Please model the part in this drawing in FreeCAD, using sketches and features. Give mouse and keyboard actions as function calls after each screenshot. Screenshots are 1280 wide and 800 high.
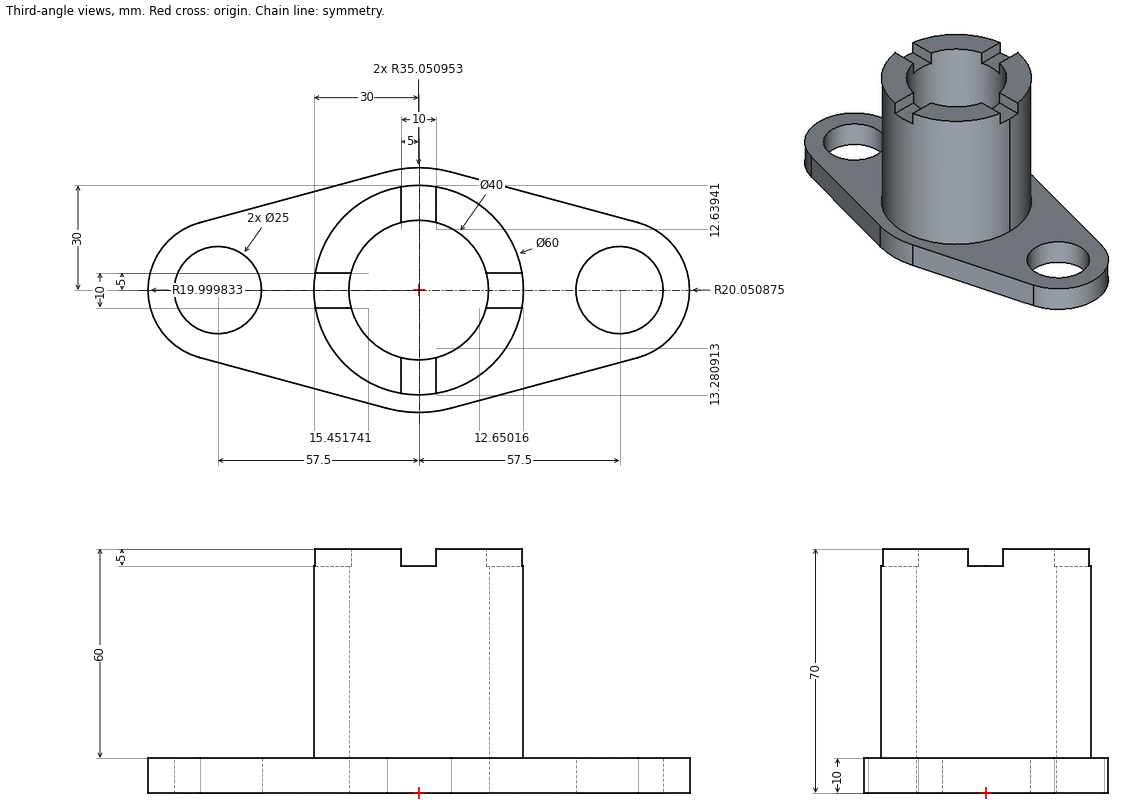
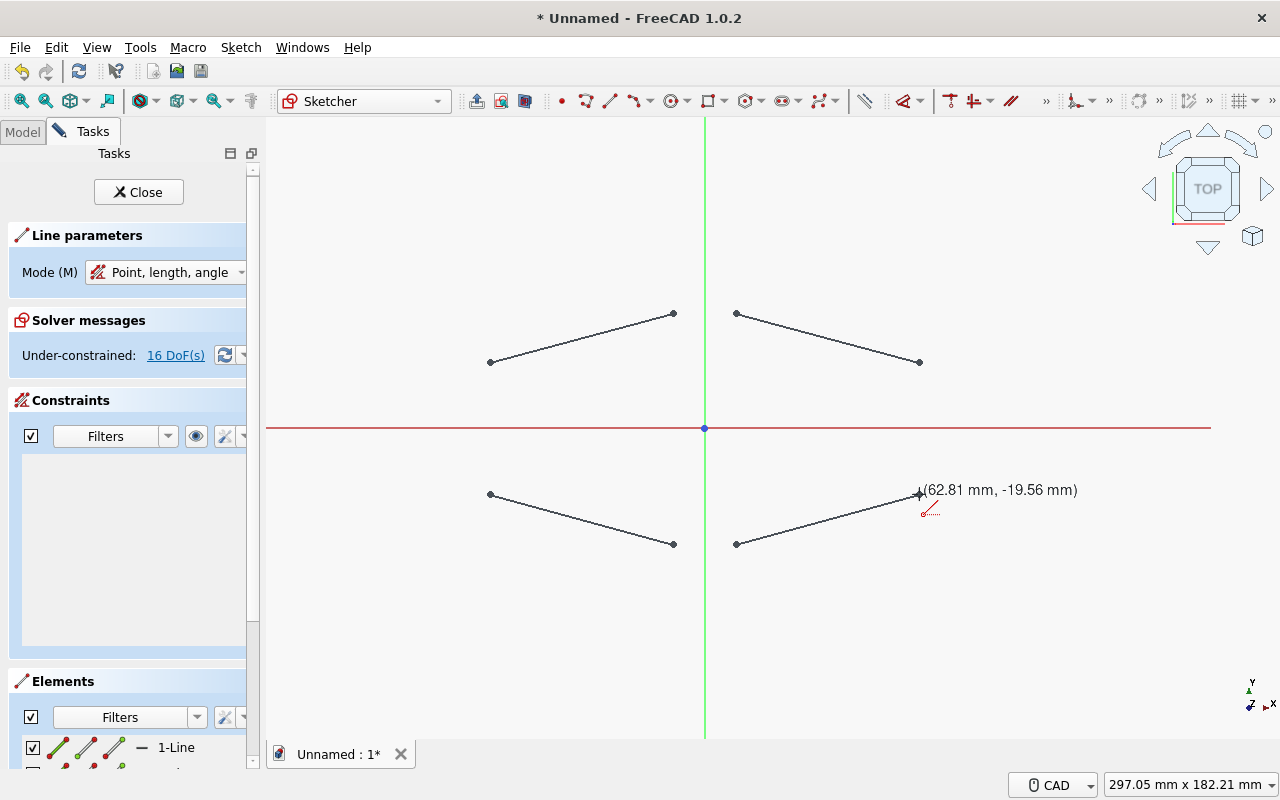
key(g)
key(3)
key(a)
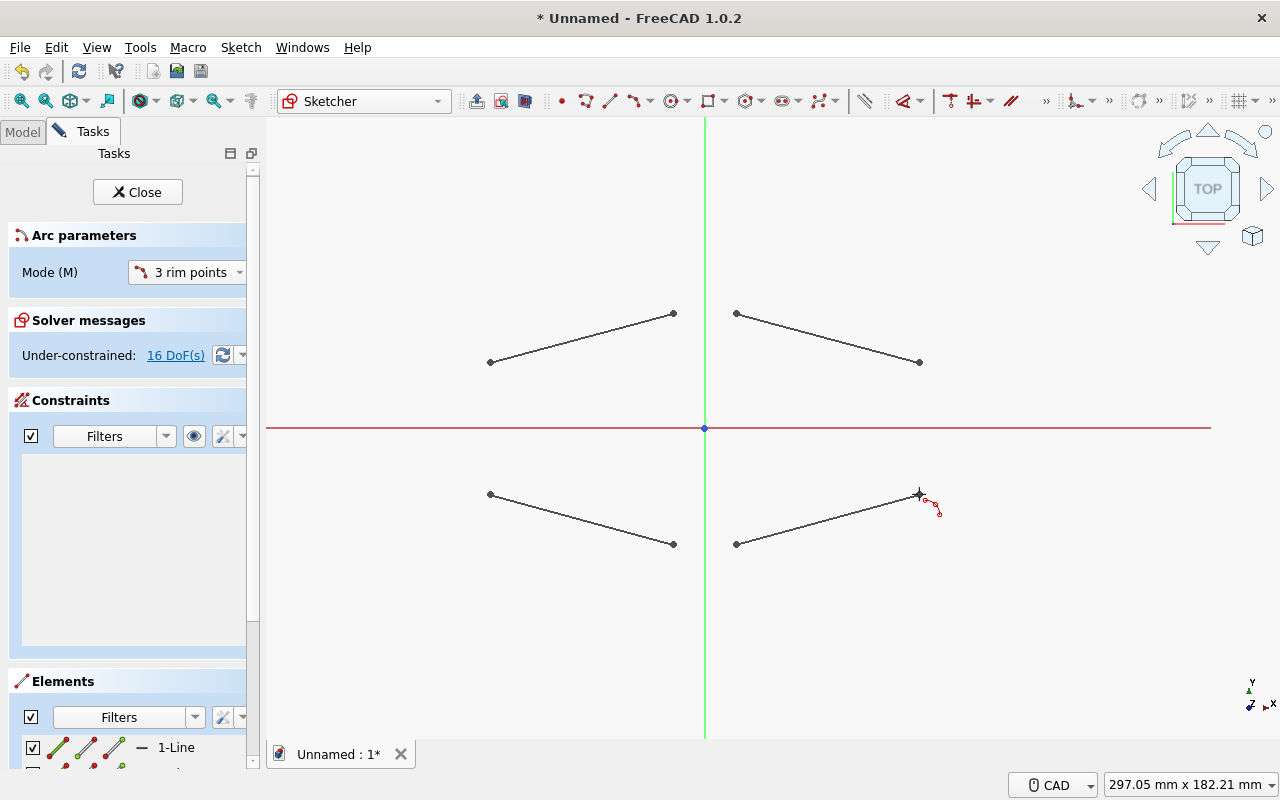
click(736, 314)
click(673, 314)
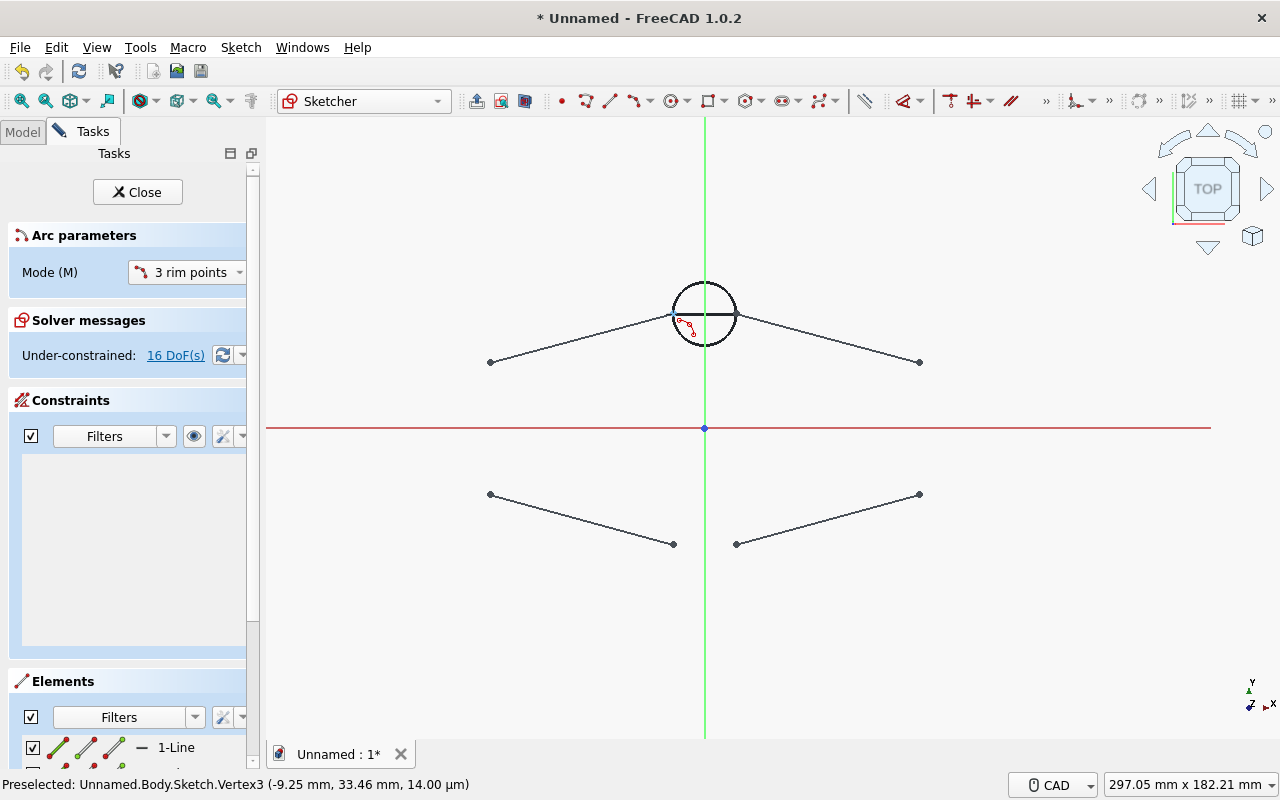
scroll(698, 309, up, 7)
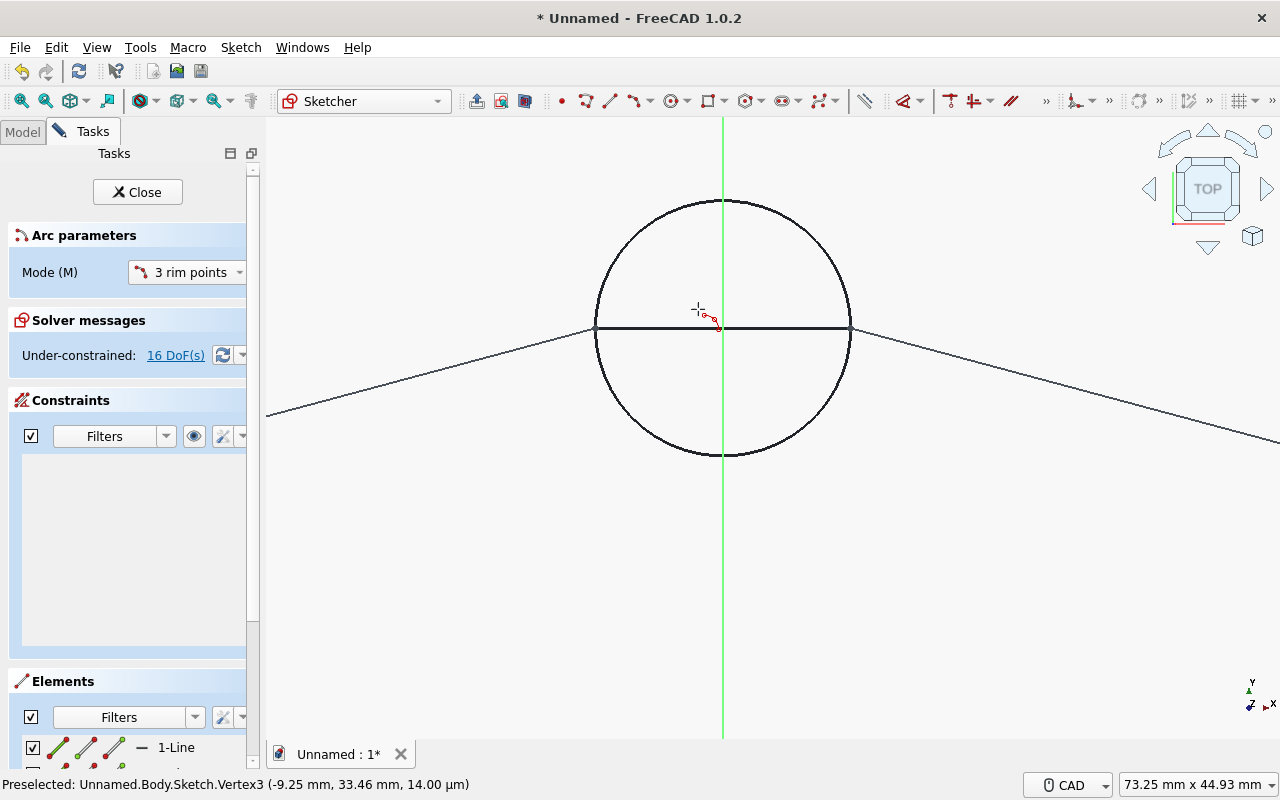
click(698, 307)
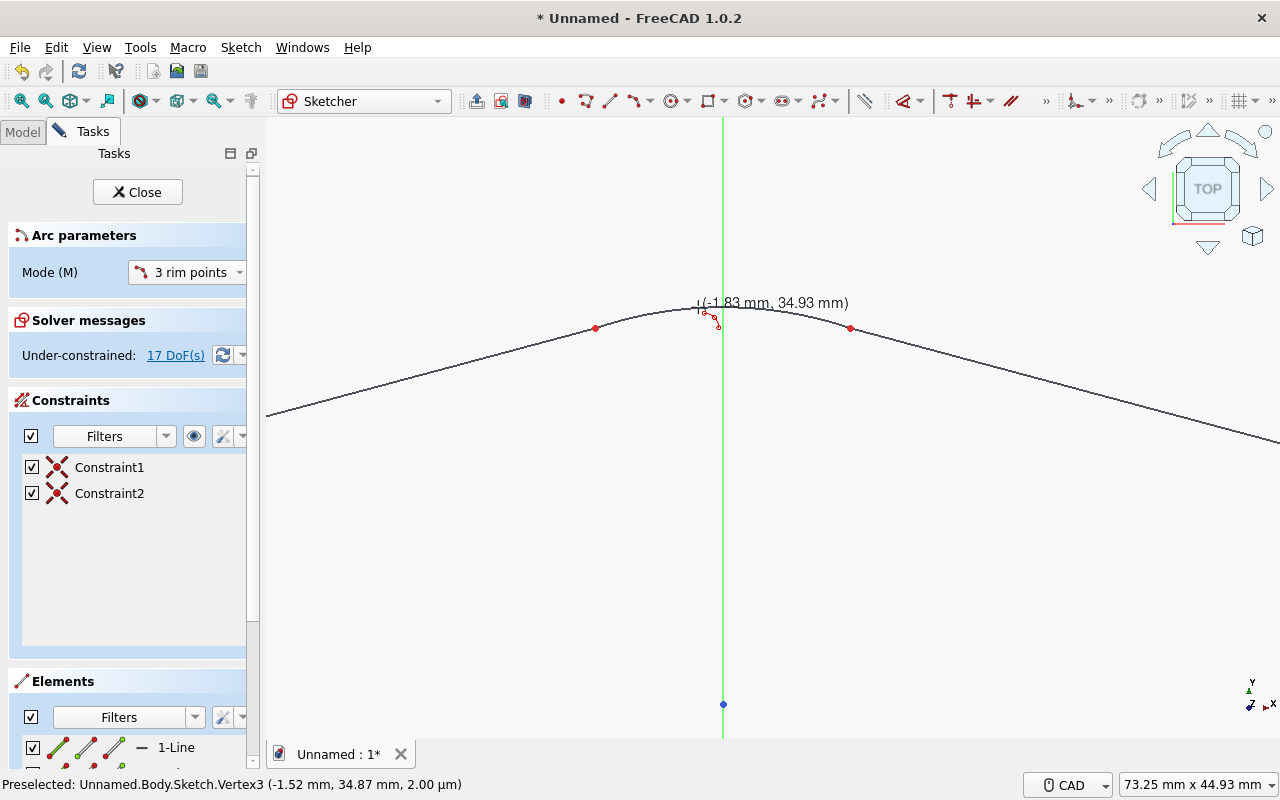
scroll(698, 309, down, 7)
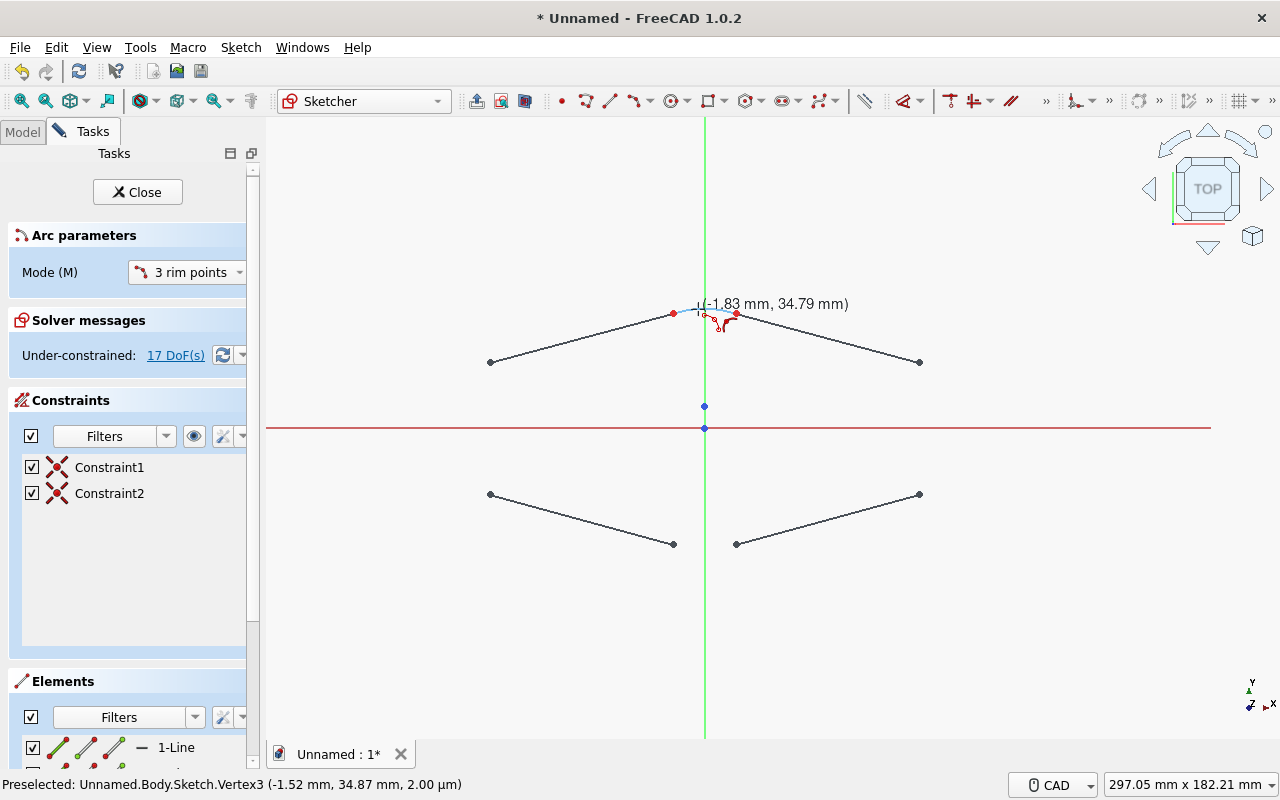
click(490, 363)
click(490, 495)
click(442, 411)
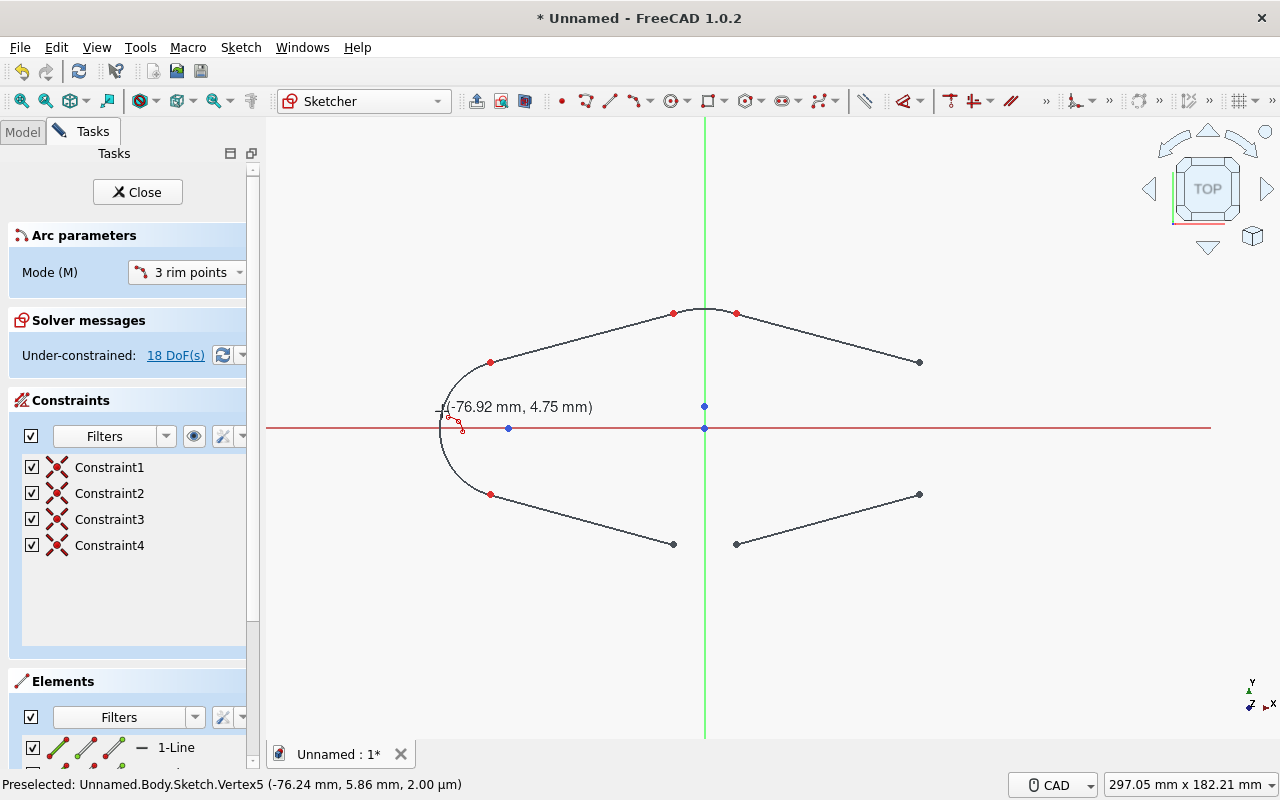
click(673, 545)
click(736, 545)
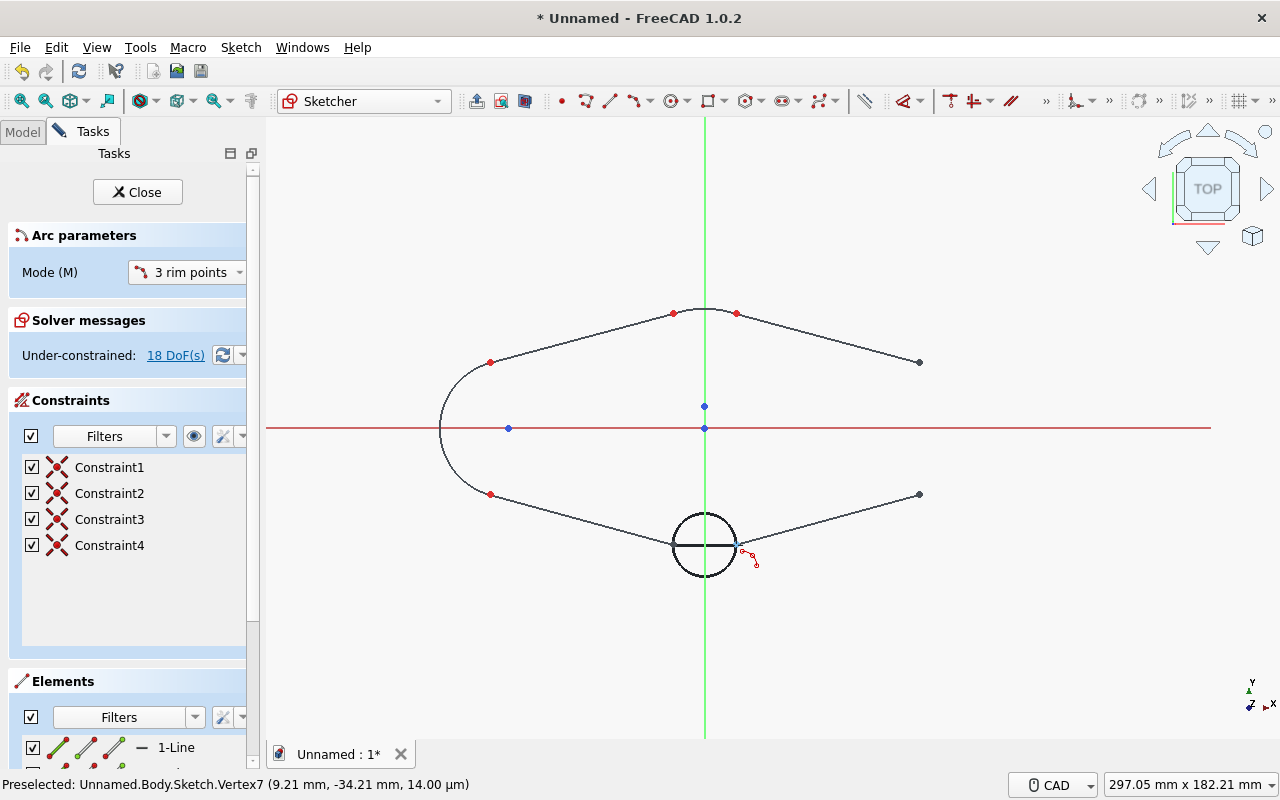
scroll(698, 548, up, 7)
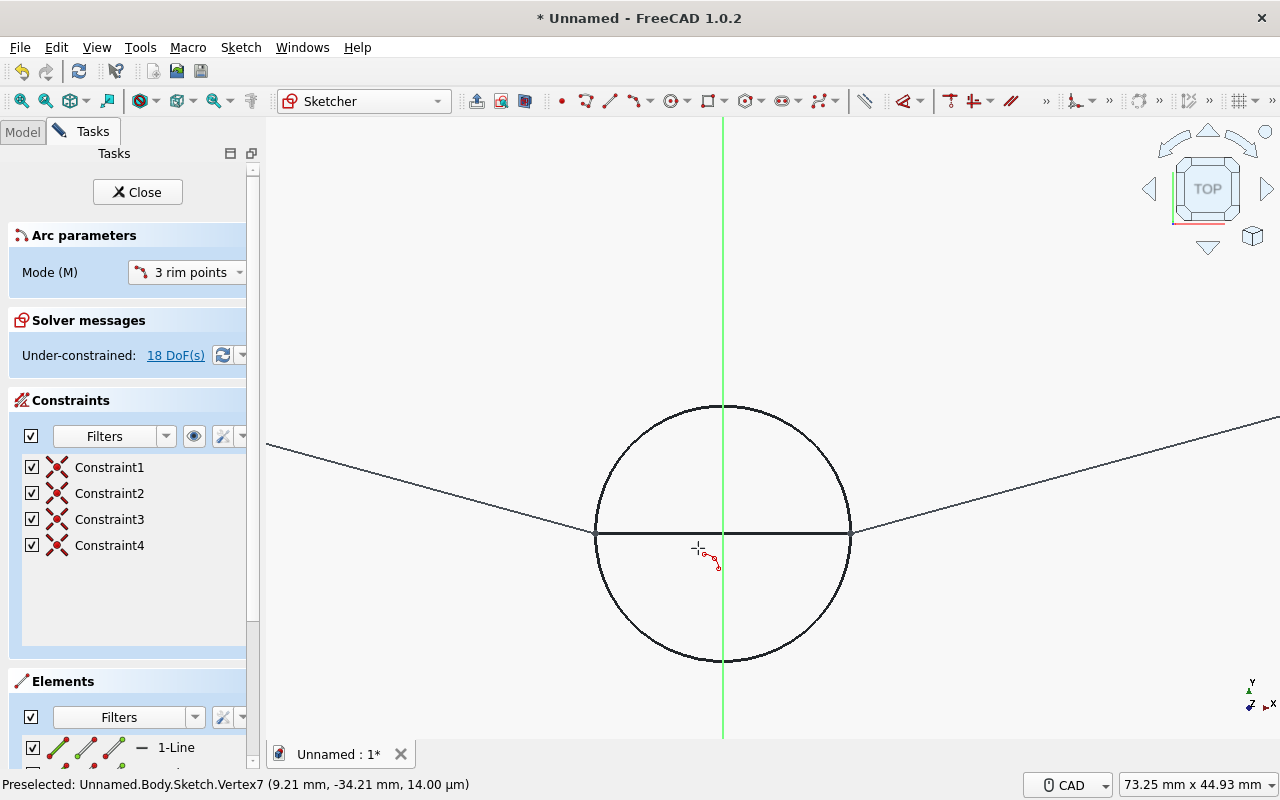
click(698, 545)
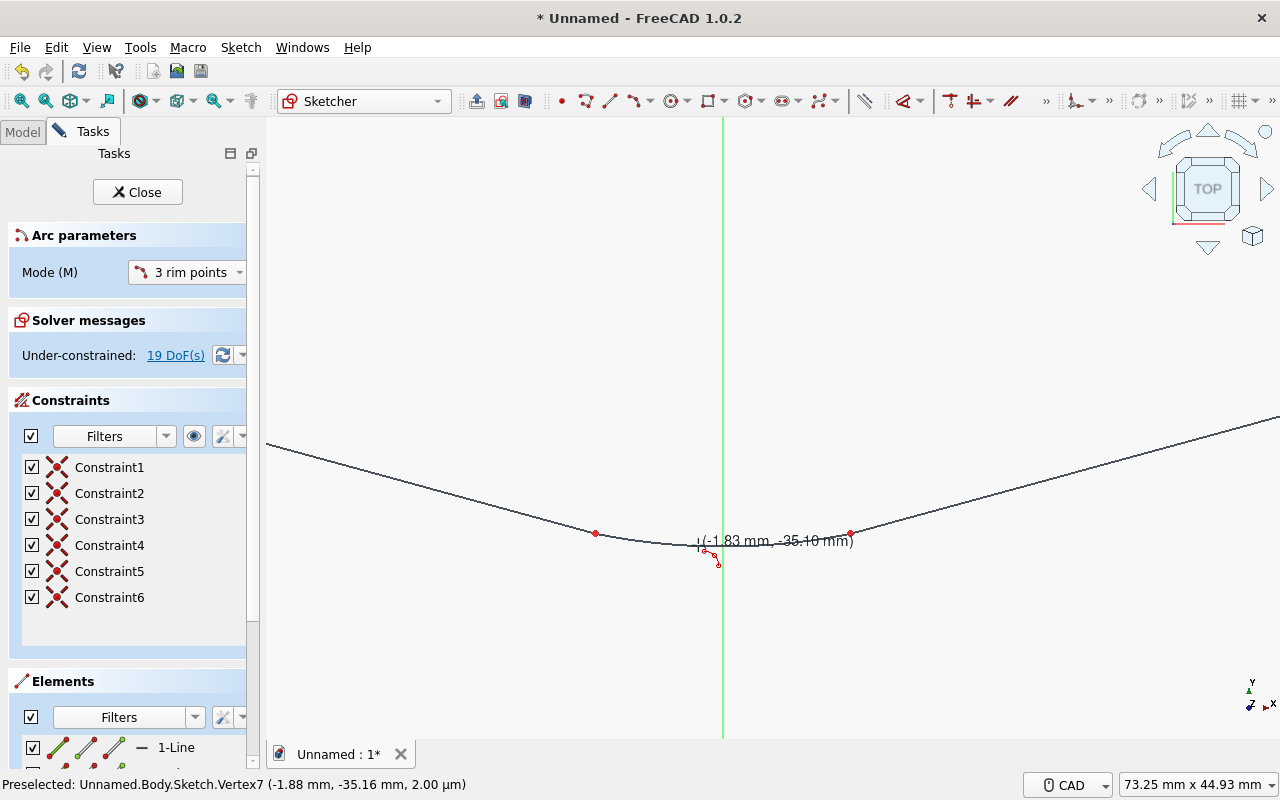
scroll(698, 548, down, 7)